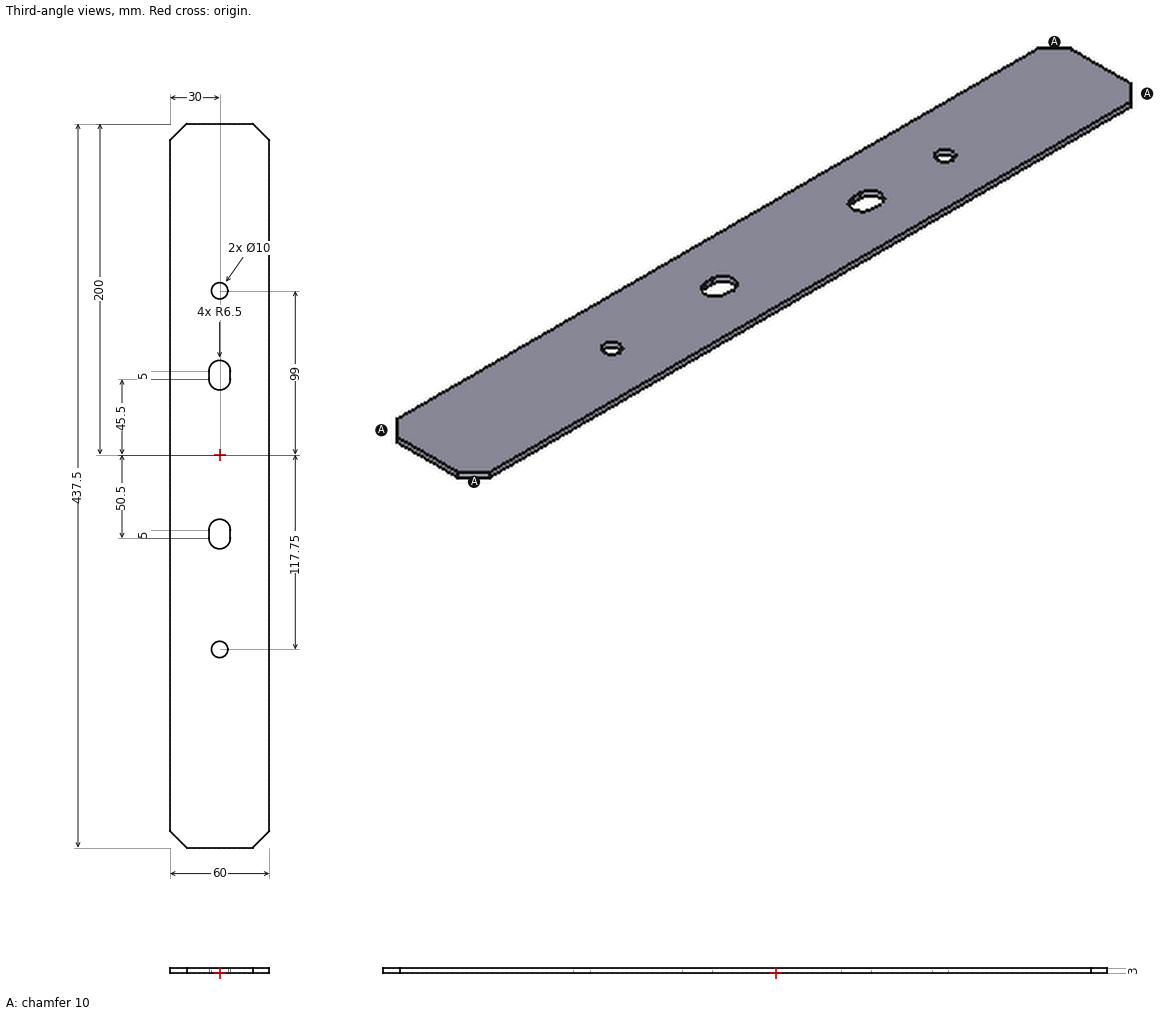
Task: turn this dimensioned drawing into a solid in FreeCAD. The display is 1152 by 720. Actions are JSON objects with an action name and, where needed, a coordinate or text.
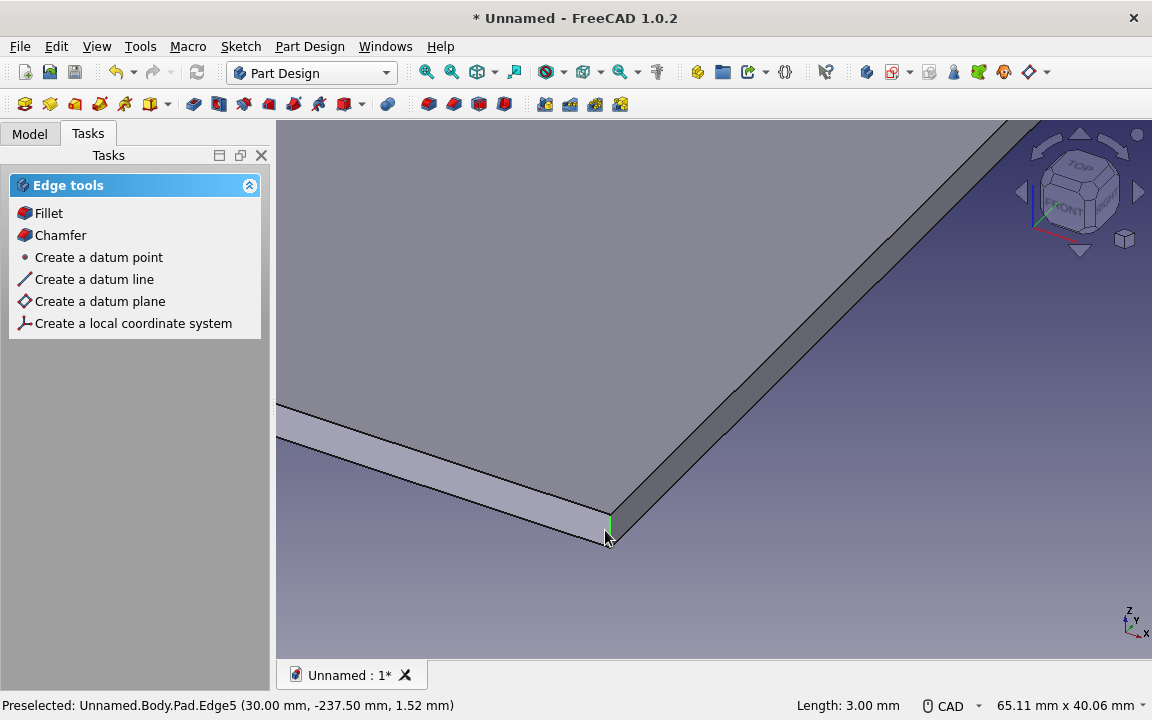
{"action": "left_click", "coordinate": [427, 72]}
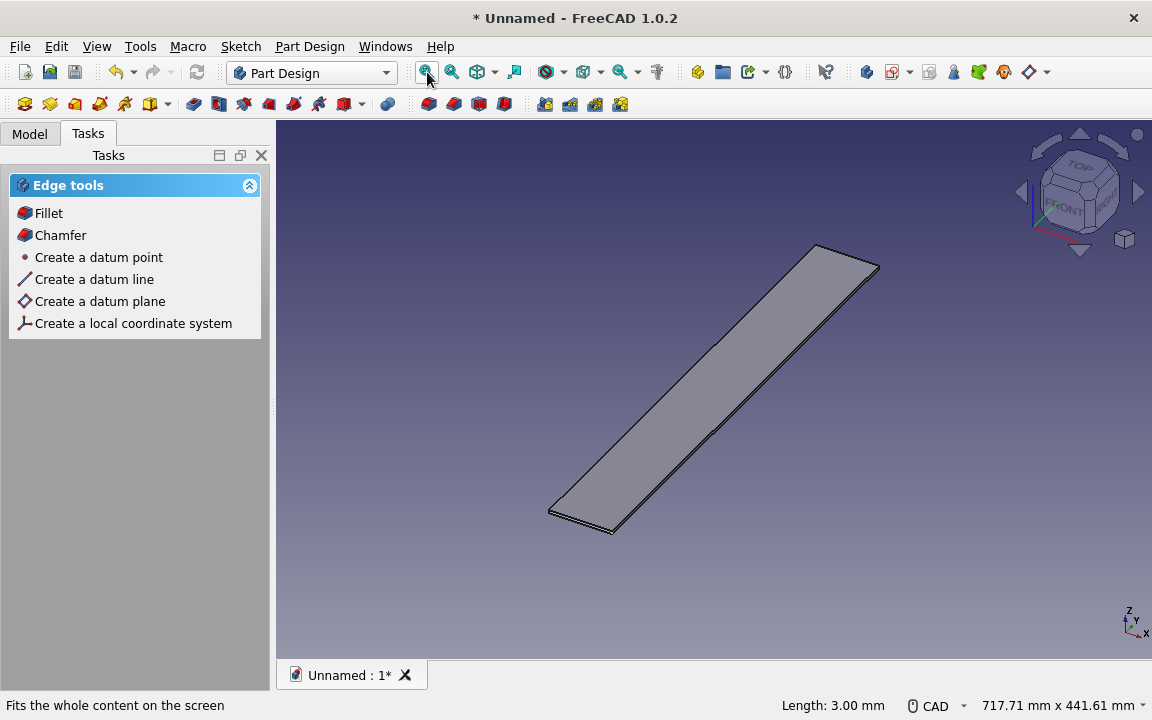
{"action": "key", "text": "0"}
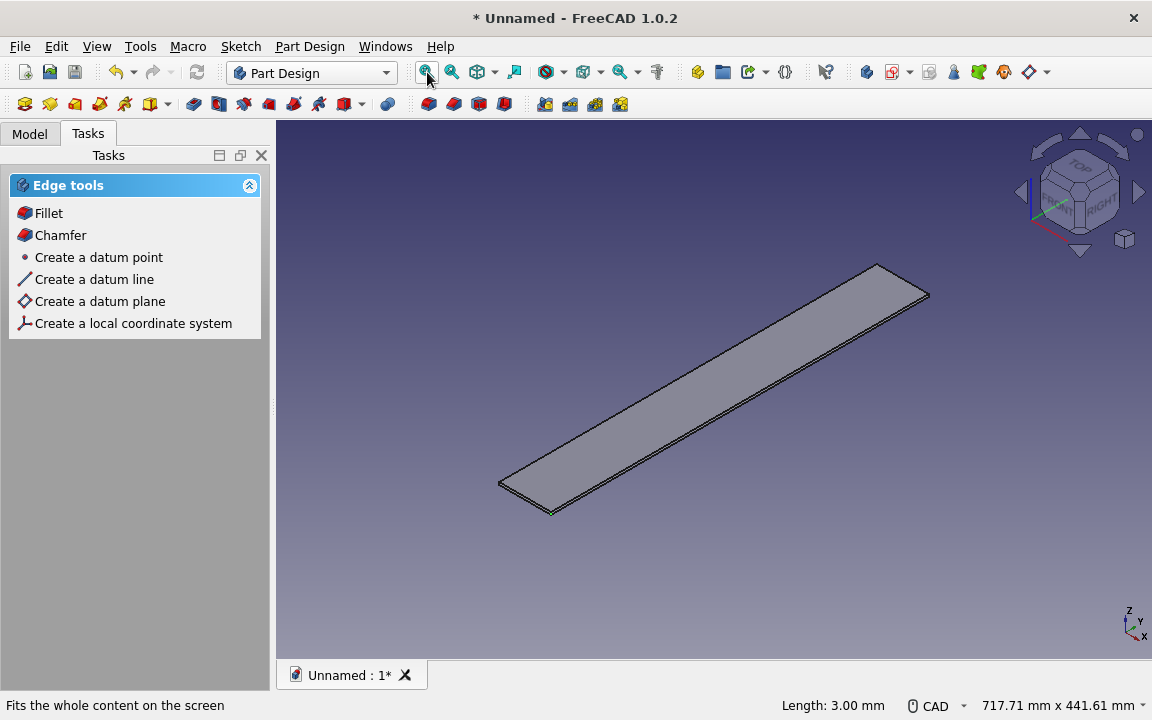
{"action": "scroll", "coordinate": [499, 483], "scroll_direction": "up", "scroll_amount": 12}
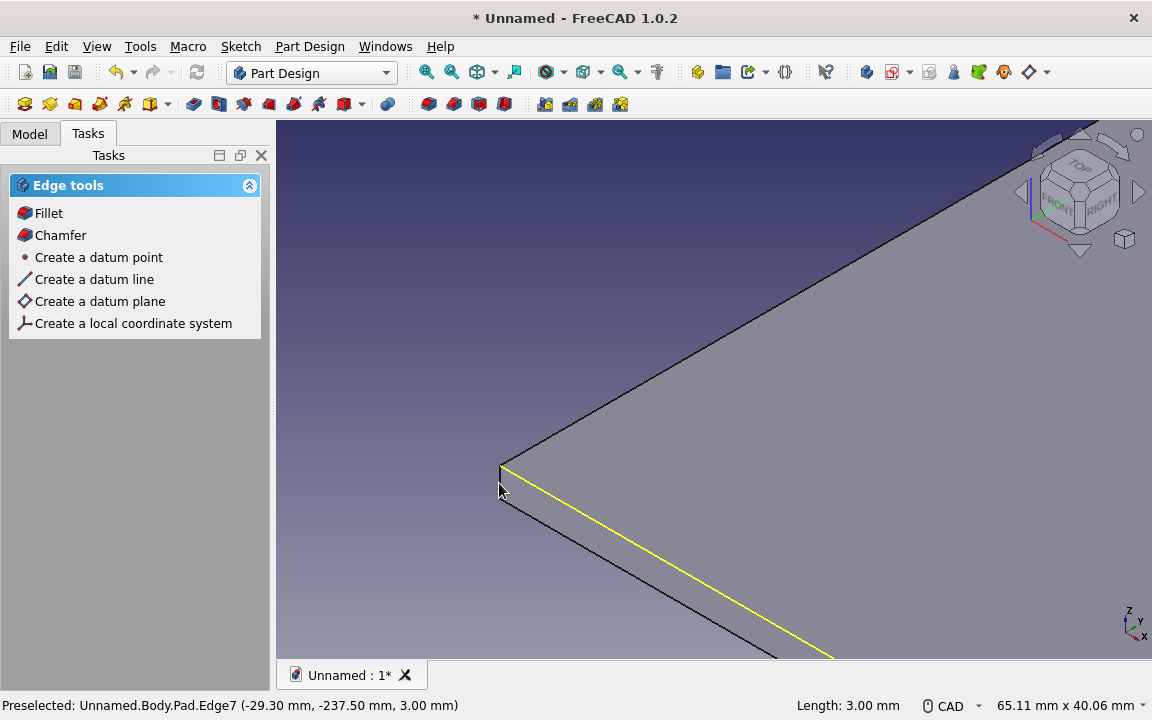
{"action": "left_click", "coordinate": [427, 72]}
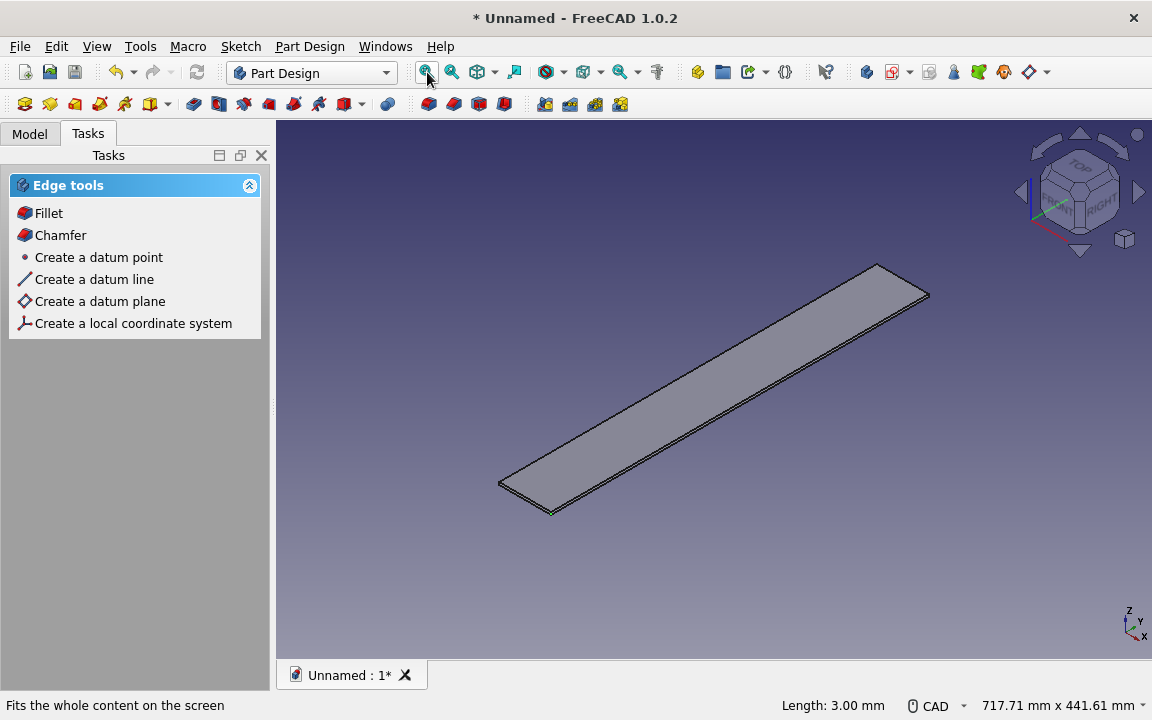
{"action": "key", "text": "2"}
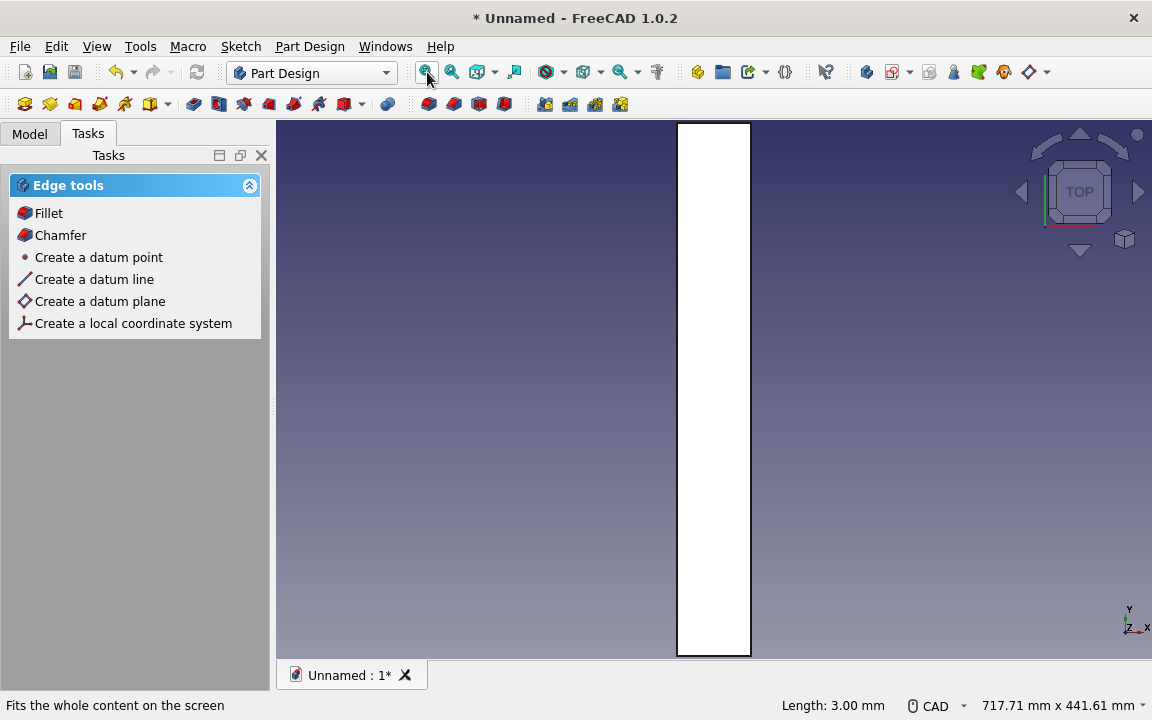
{"action": "key", "text": "1"}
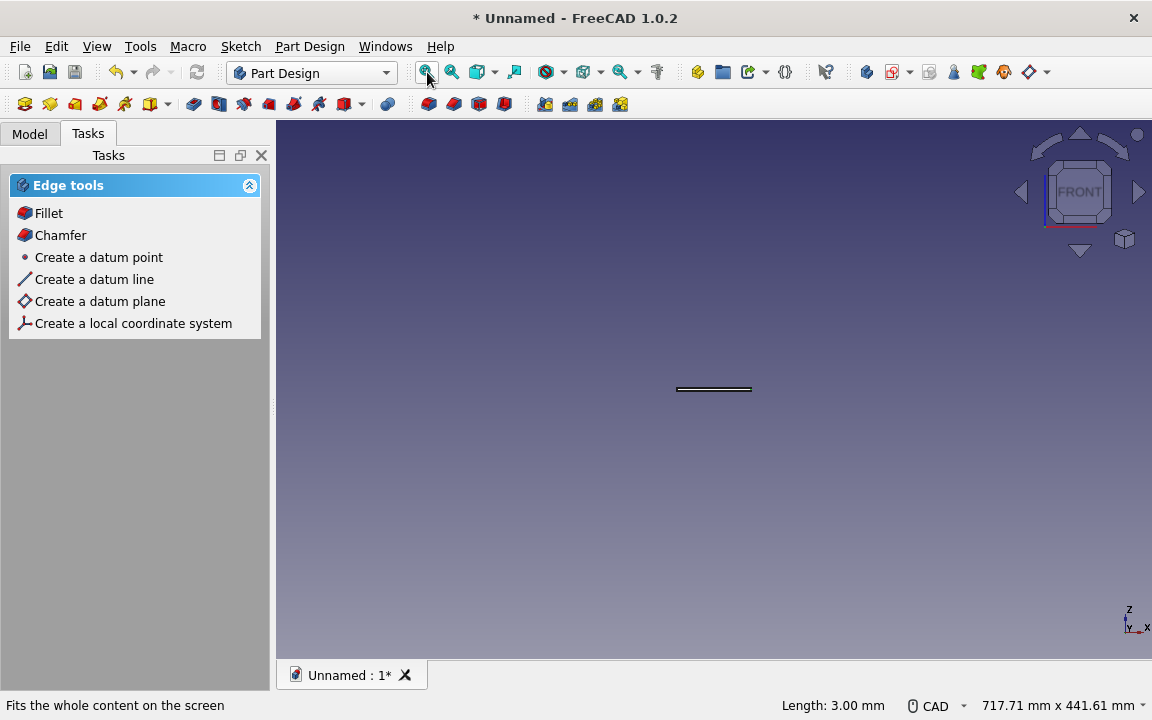
{"action": "left_click", "coordinate": [427, 72]}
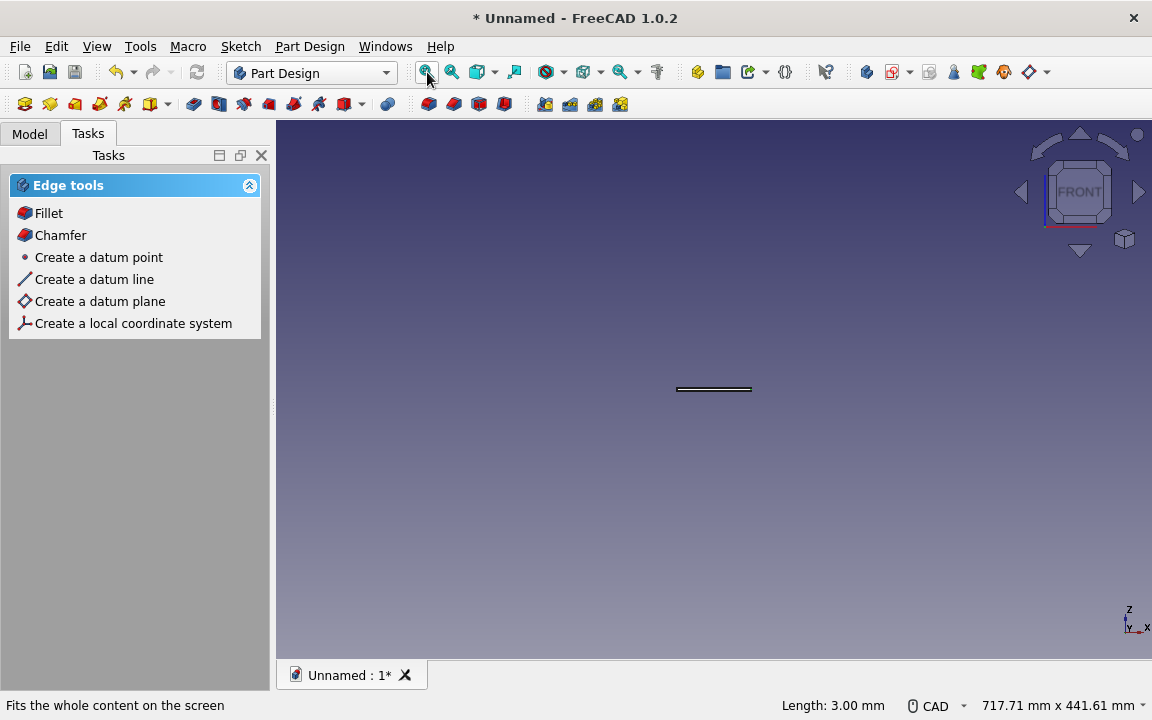
{"action": "scroll", "coordinate": [677, 389], "scroll_direction": "up", "scroll_amount": 12}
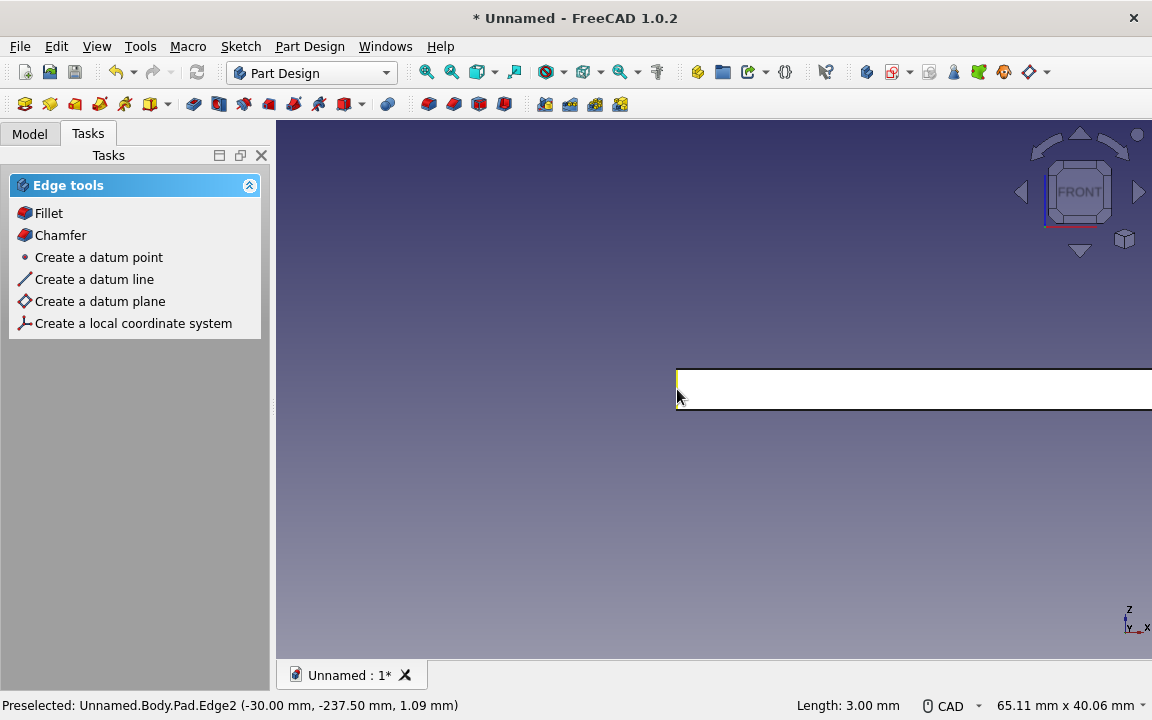
{"action": "left_click", "coordinate": [677, 389], "text": "ctrl"}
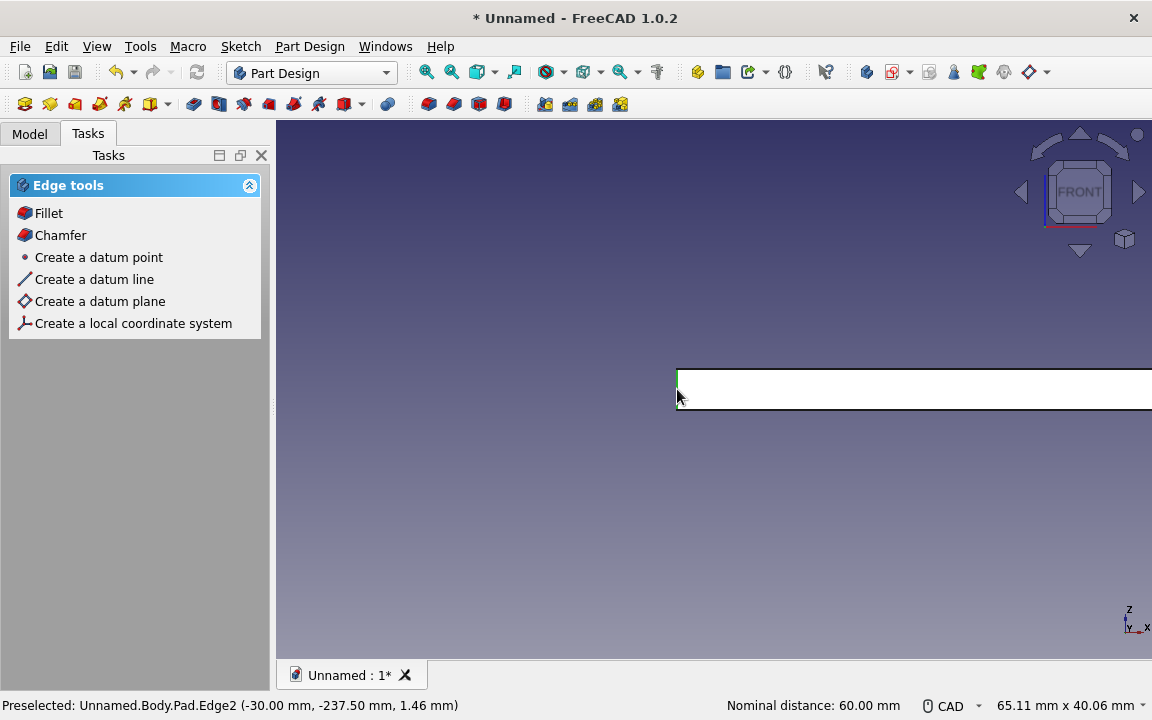
{"action": "left_click", "coordinate": [427, 72]}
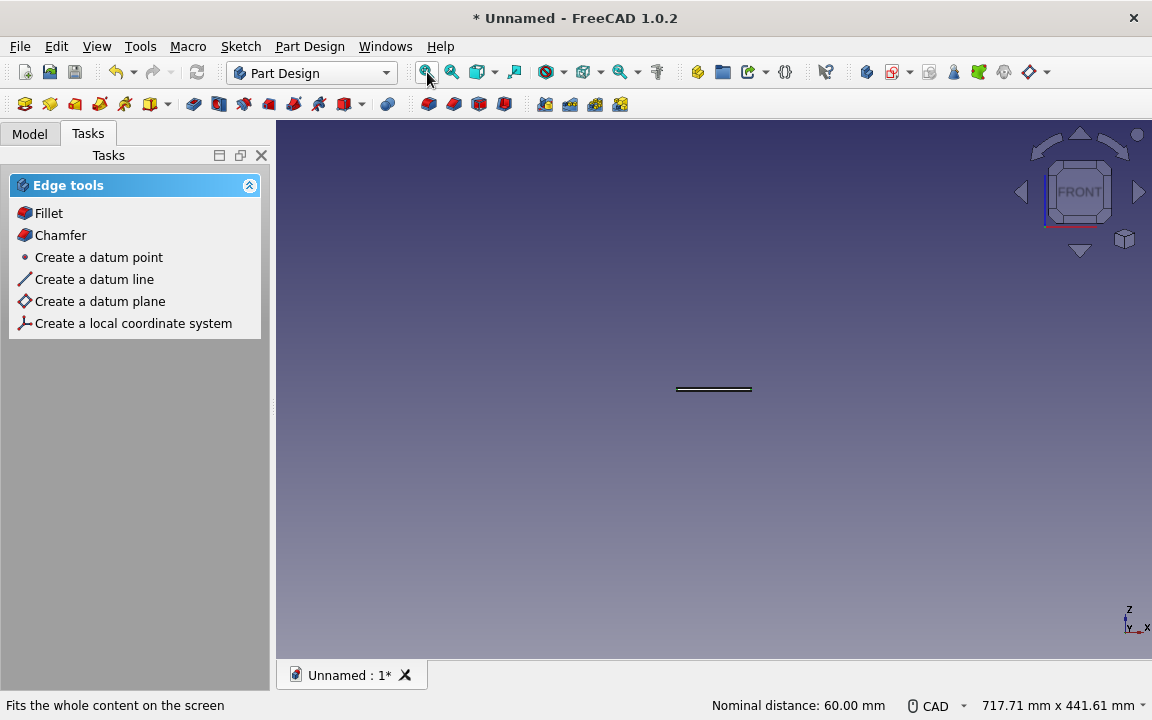
{"action": "key", "text": "3"}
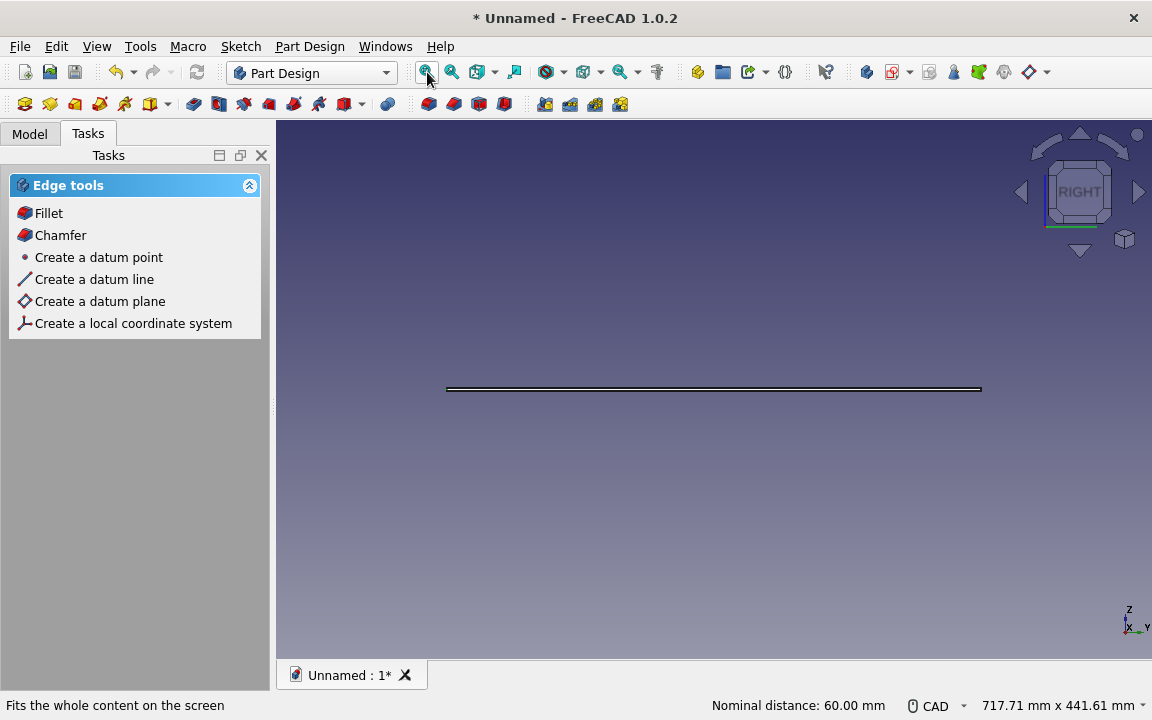
{"action": "scroll", "coordinate": [981, 388], "scroll_direction": "up", "scroll_amount": 12}